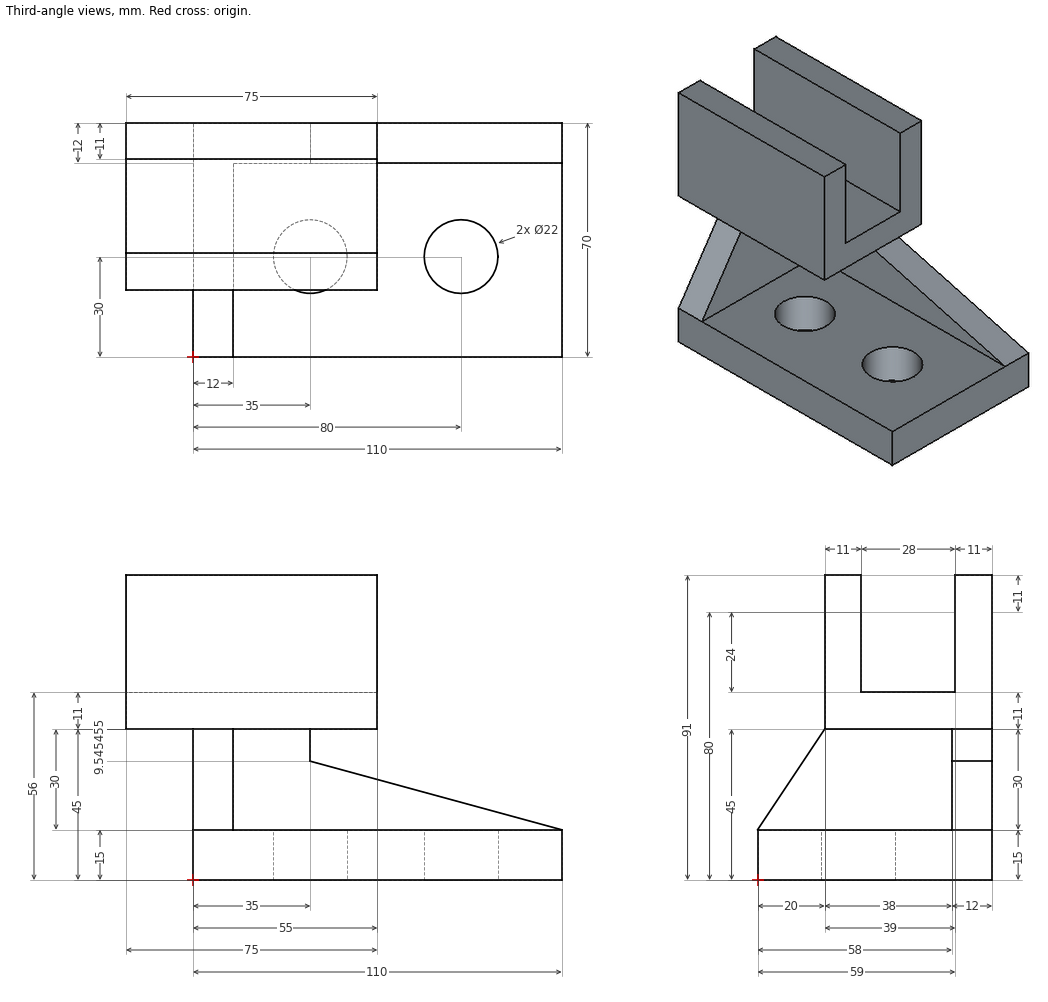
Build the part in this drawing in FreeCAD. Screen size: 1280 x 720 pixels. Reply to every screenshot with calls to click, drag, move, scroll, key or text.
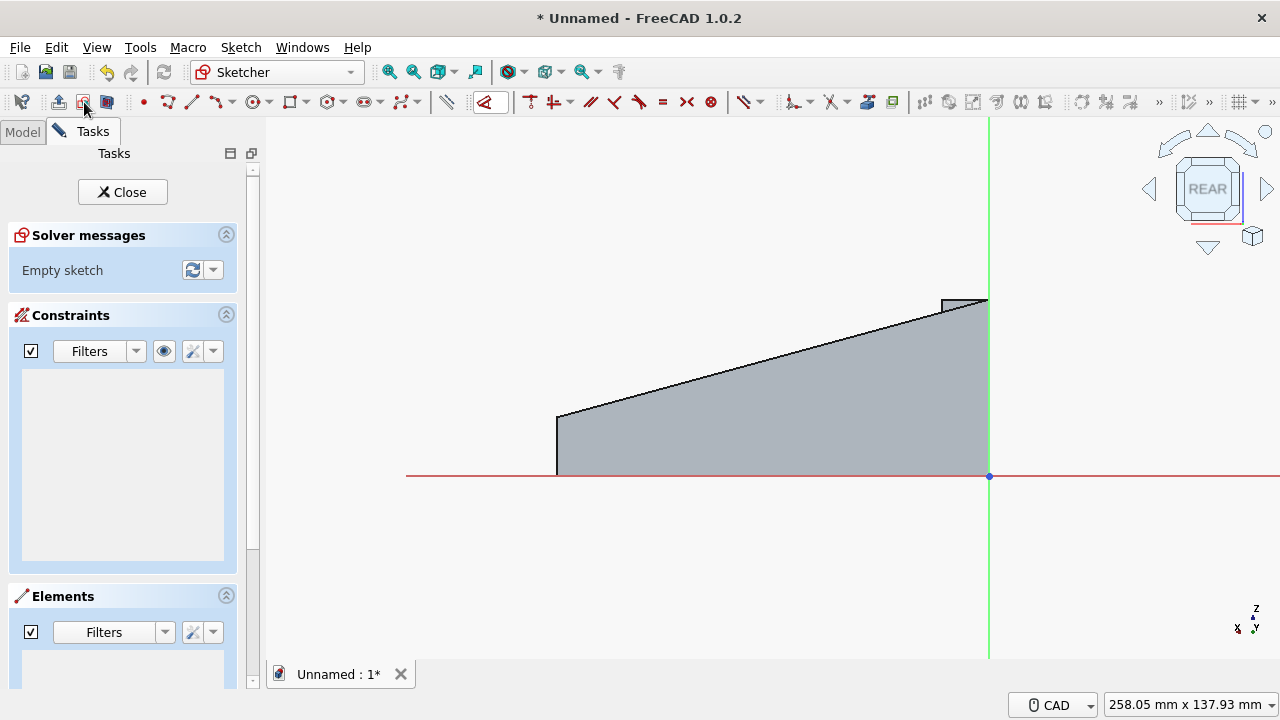
scroll(1115, 388, up, 3)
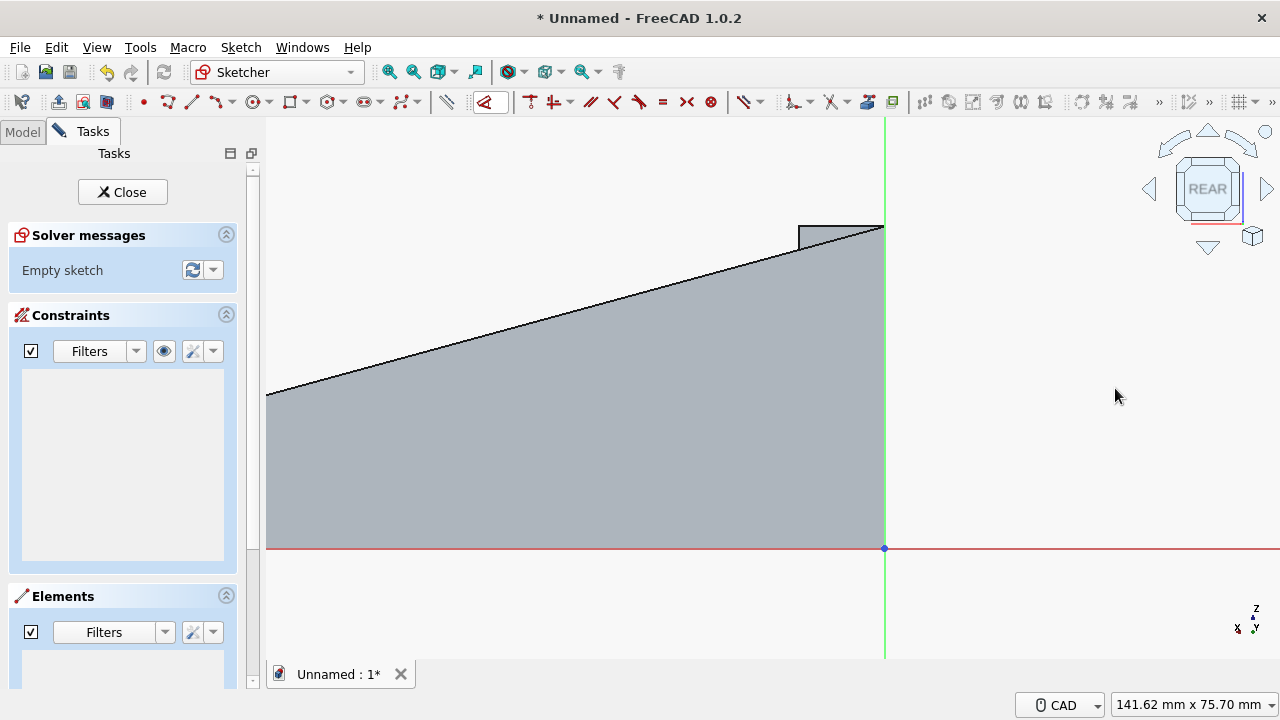
click(168, 102)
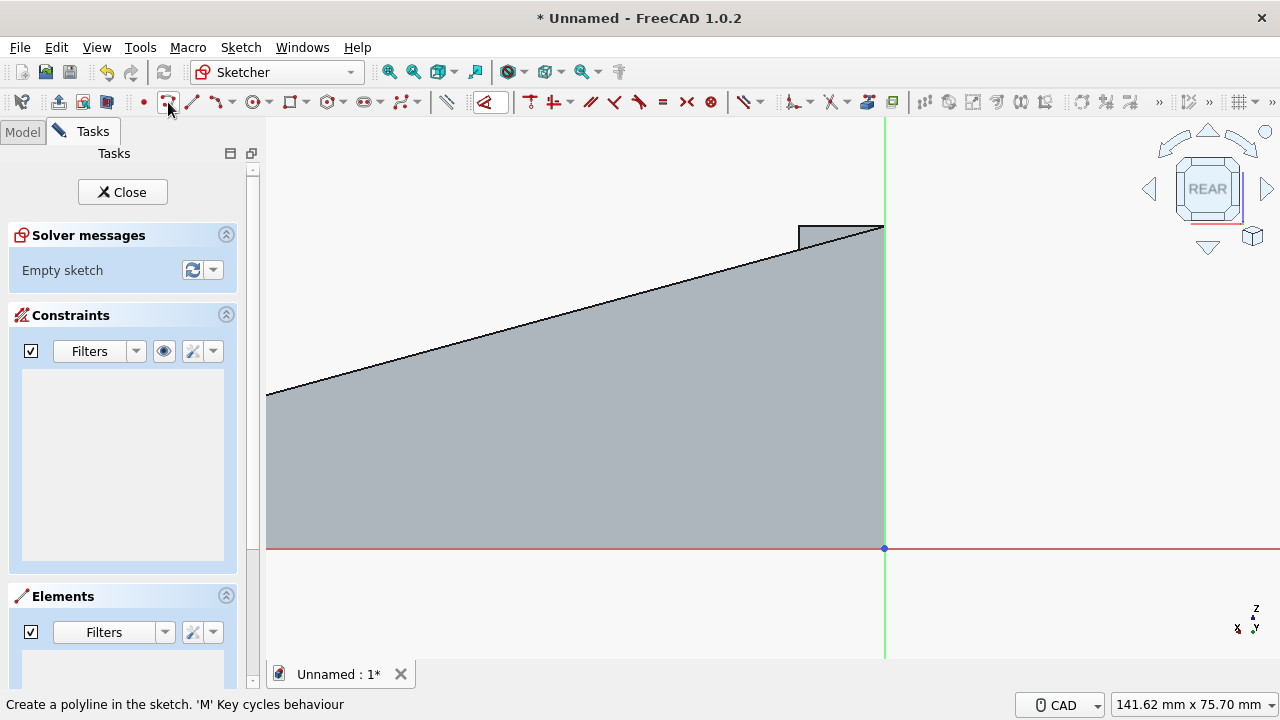
click(885, 226)
click(634, 226)
click(634, 295)
click(885, 227)
key(Escape)
key(Escape)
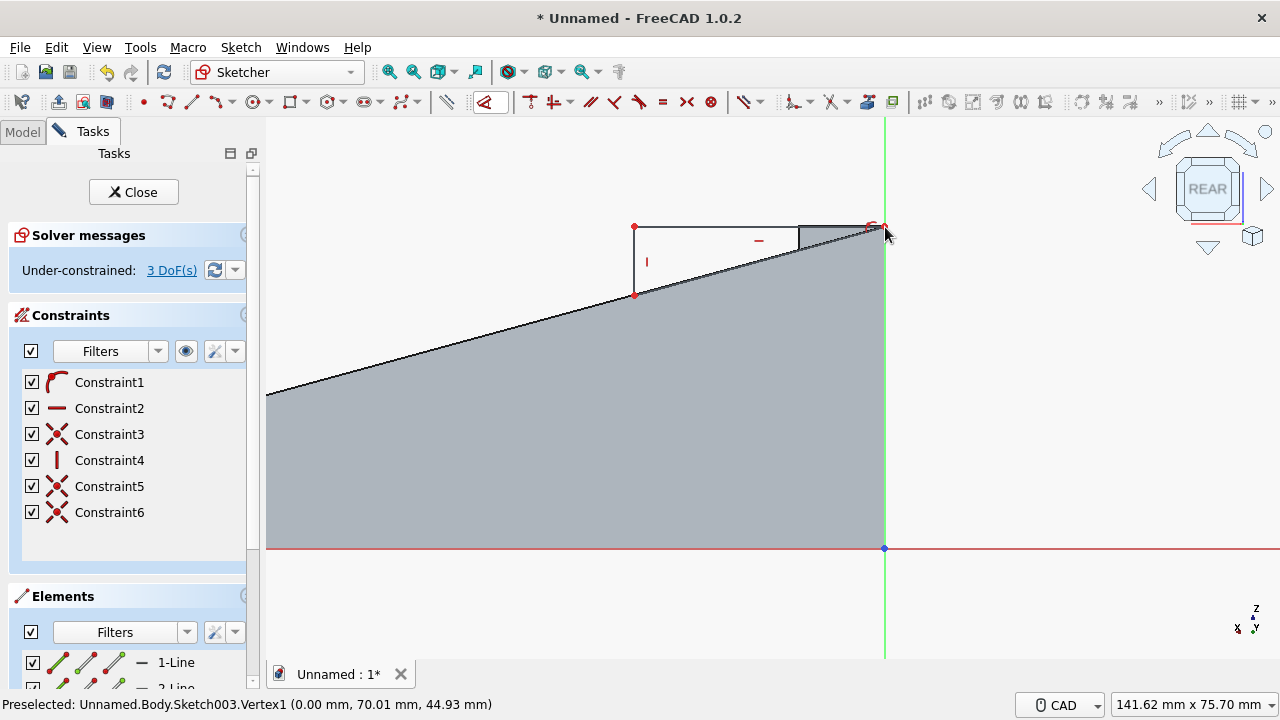
click(810, 227)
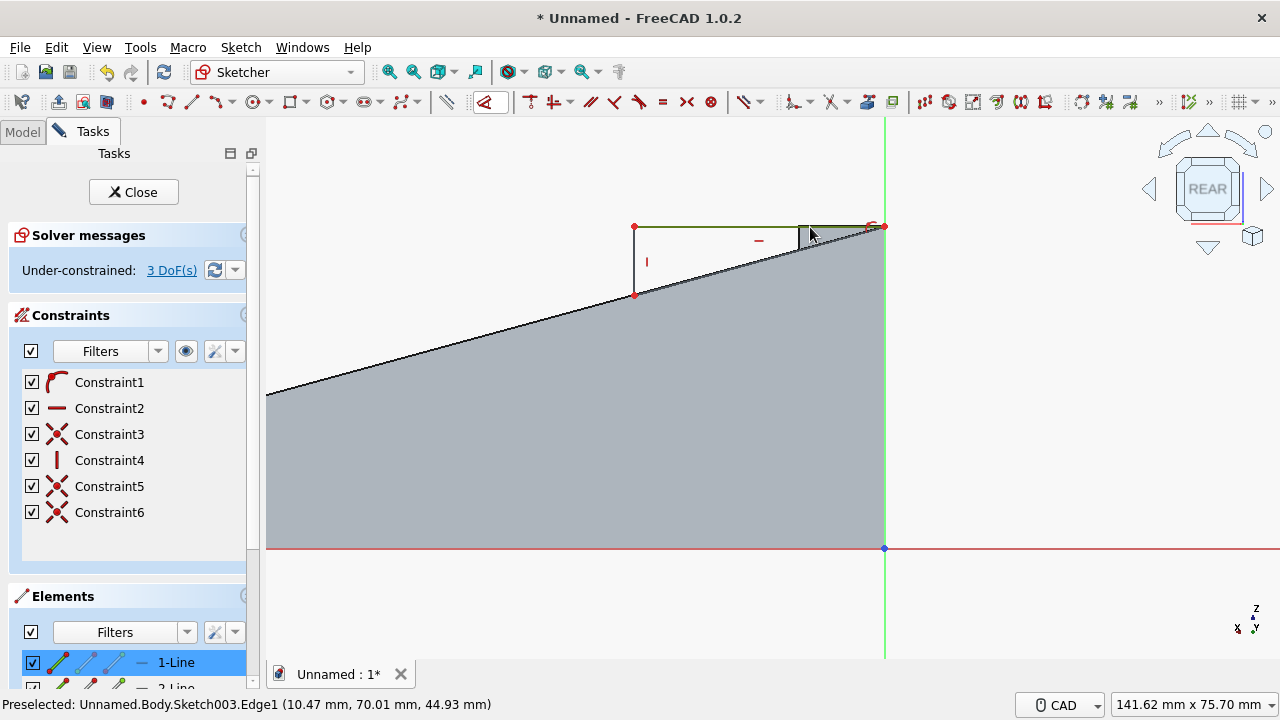
key(l)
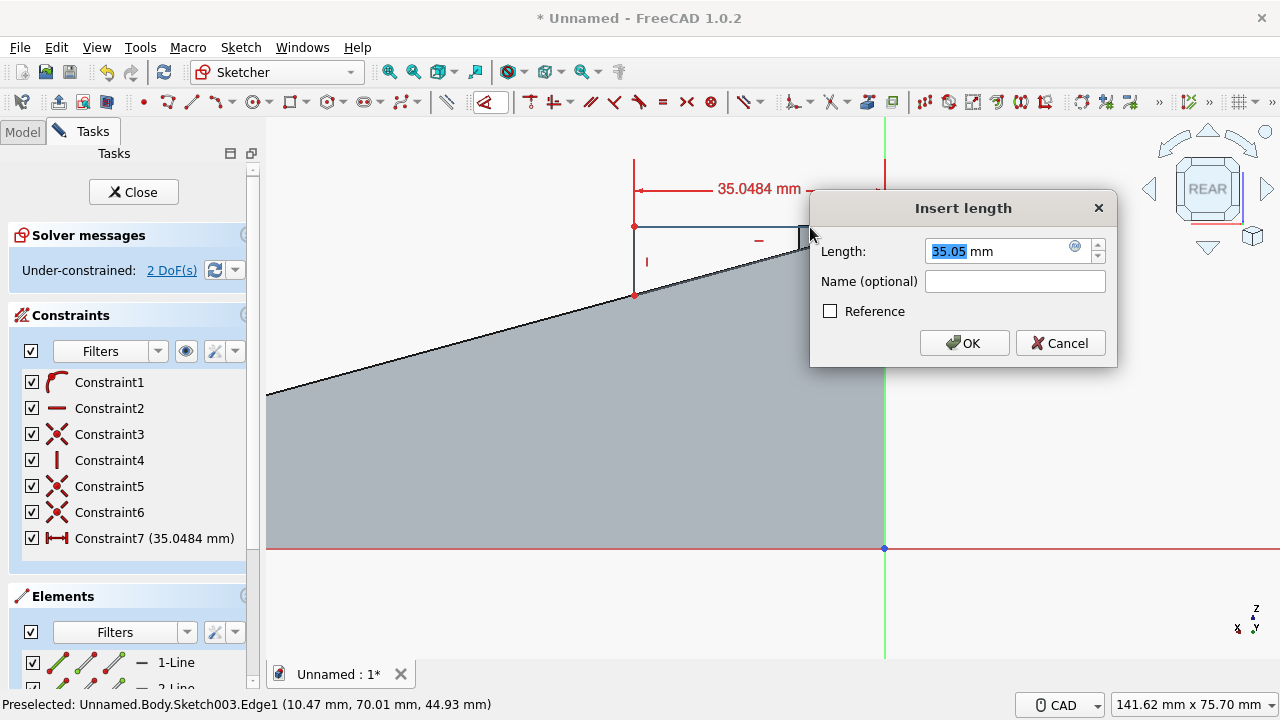
text(35)
key(Return)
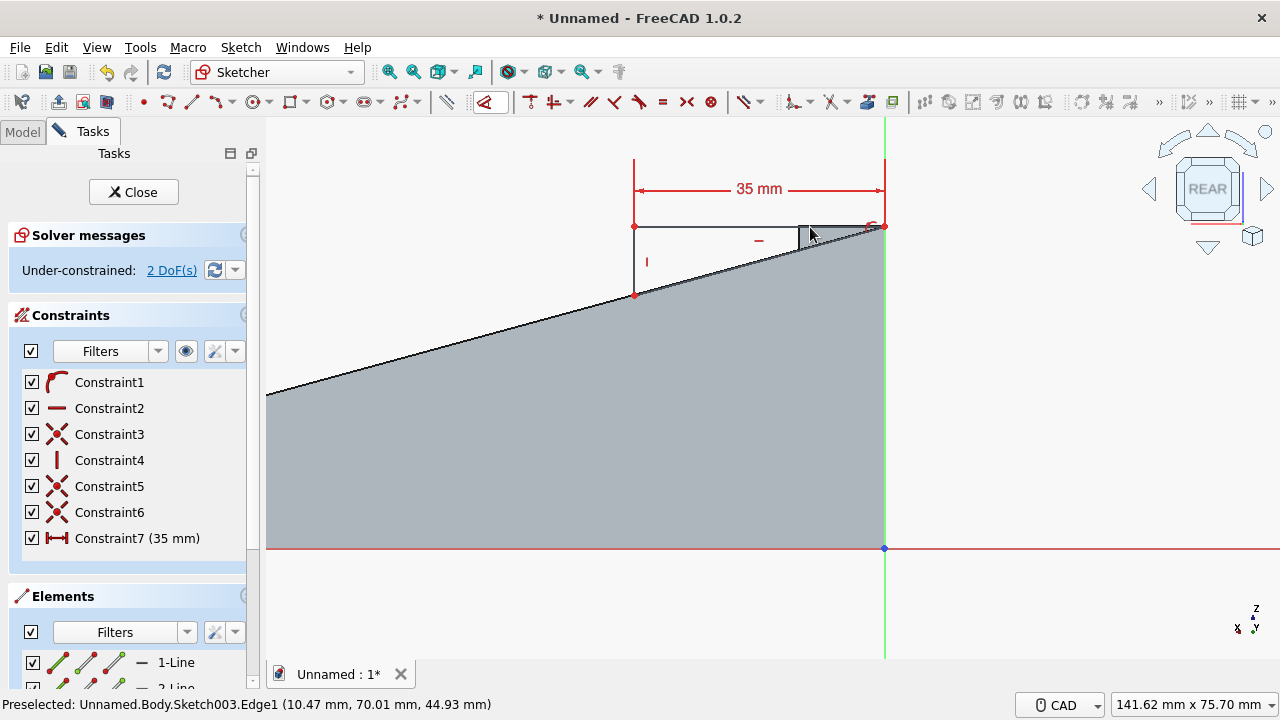
click(885, 227)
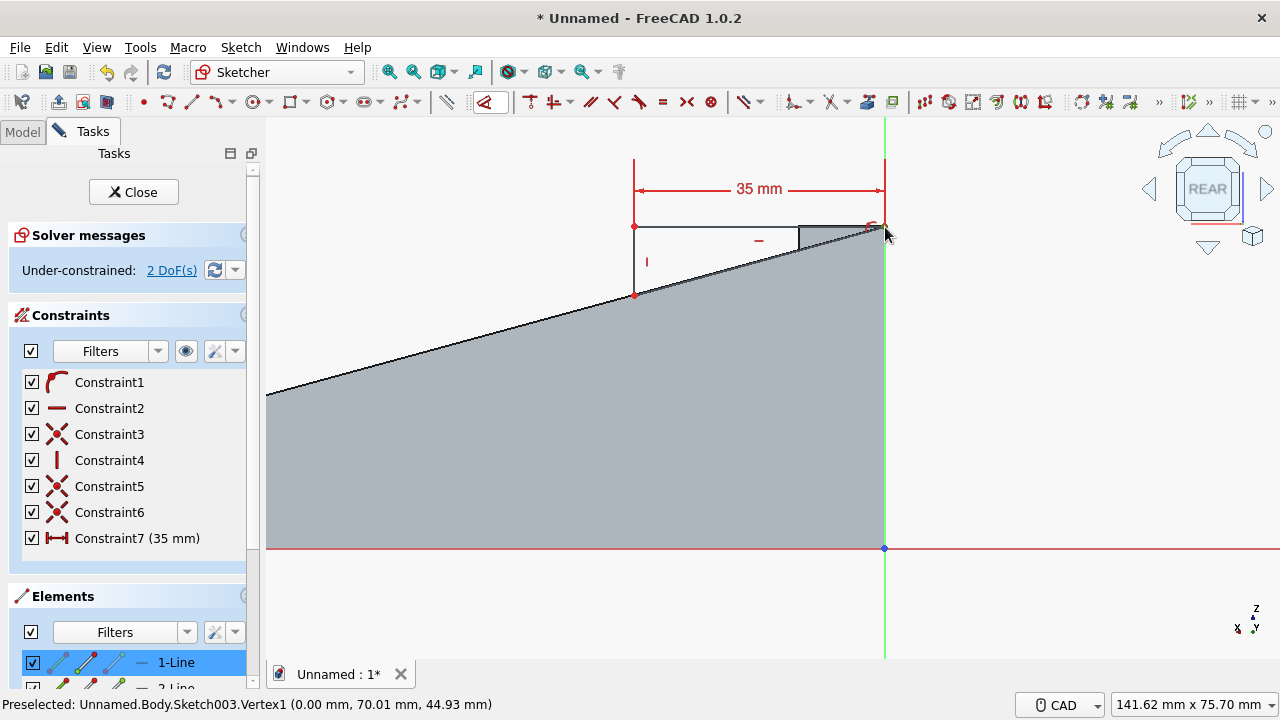
key(i)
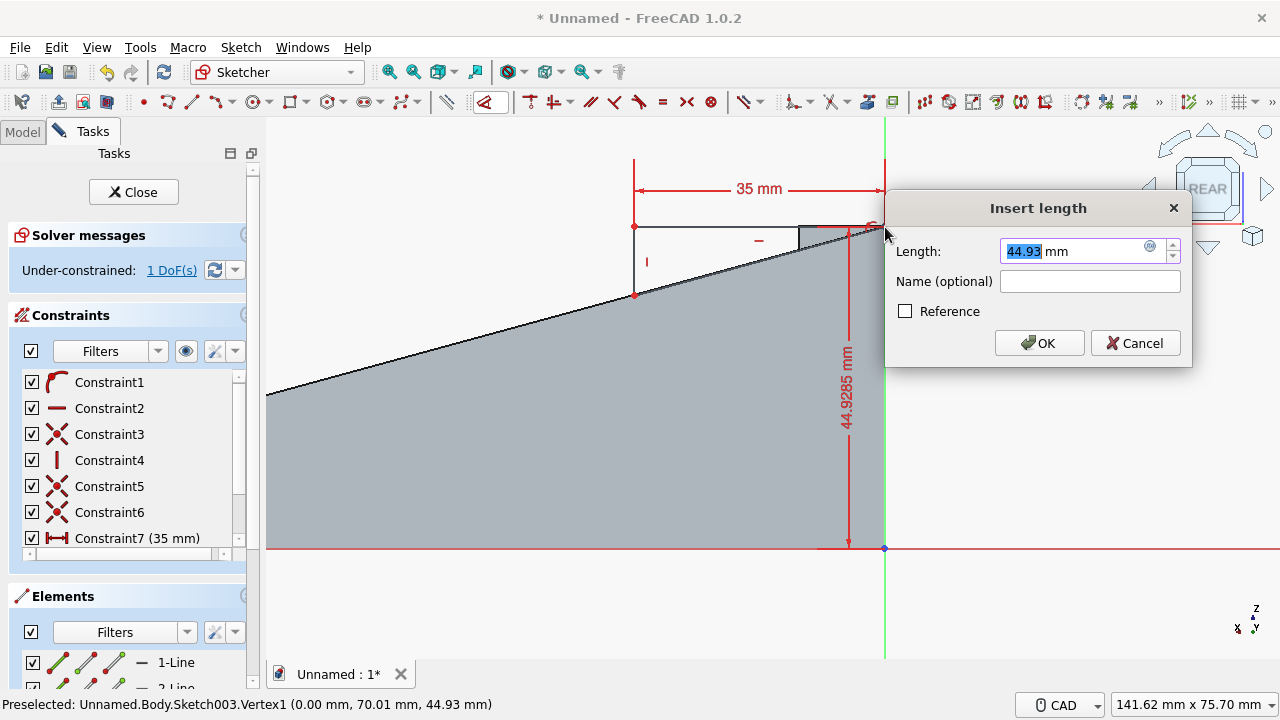
text(45)
key(Return)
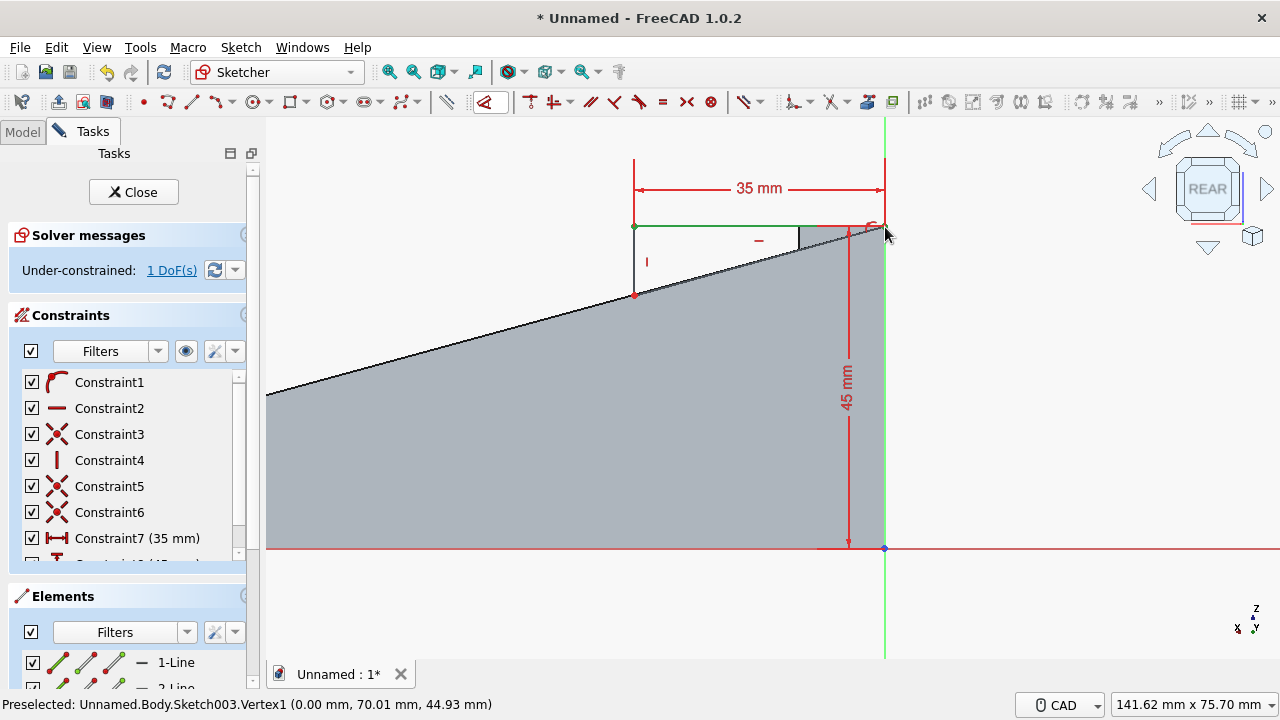
click(634, 247)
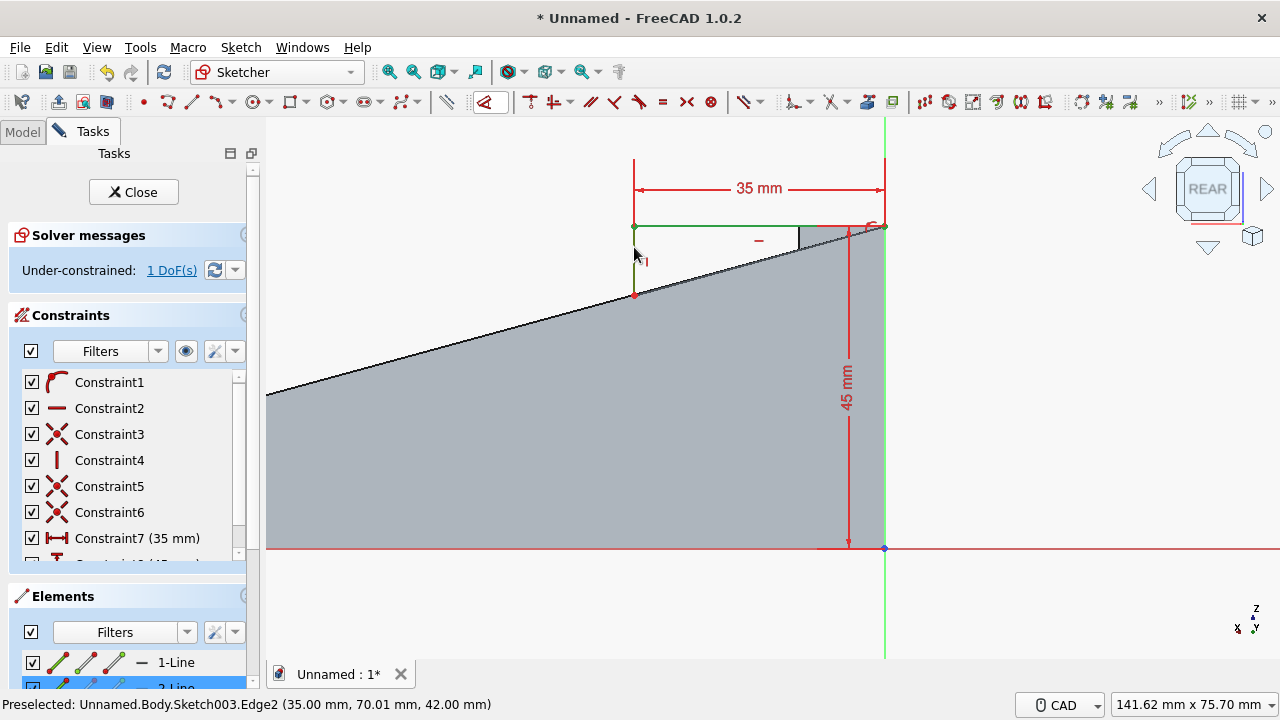
click(502, 102)